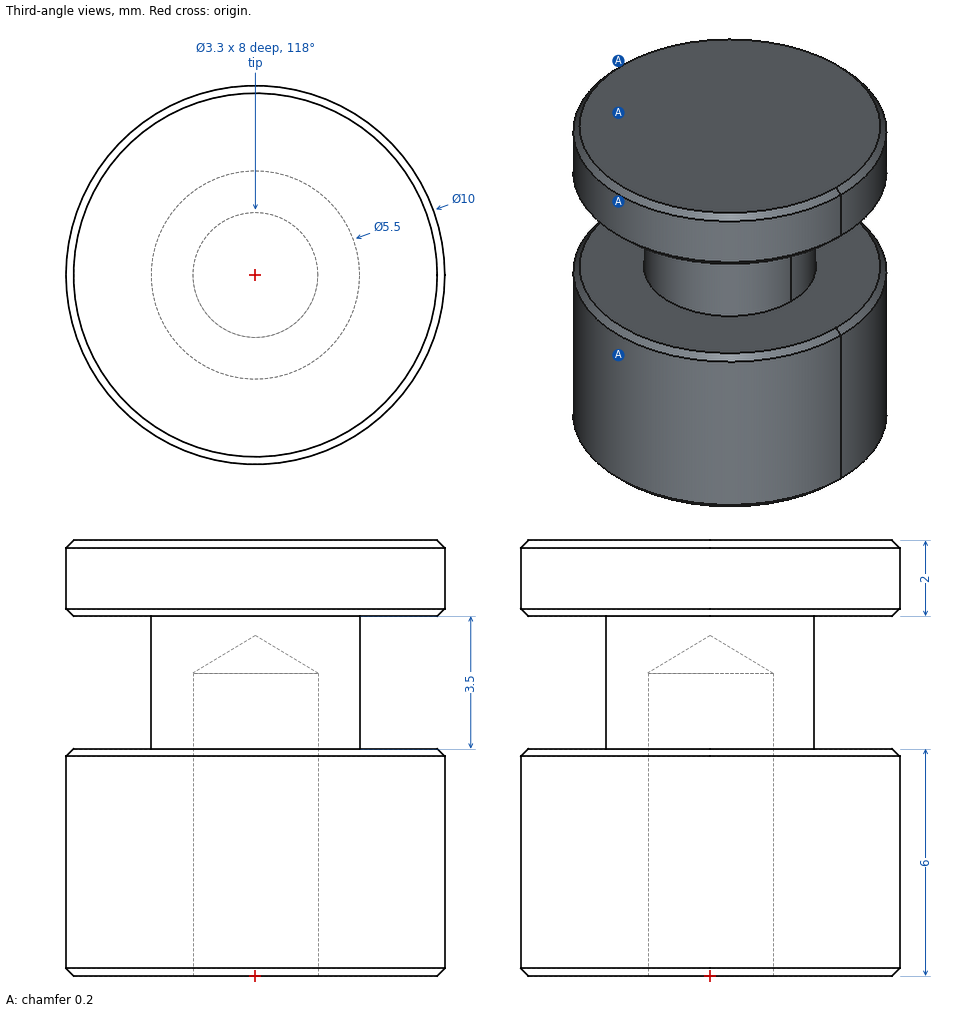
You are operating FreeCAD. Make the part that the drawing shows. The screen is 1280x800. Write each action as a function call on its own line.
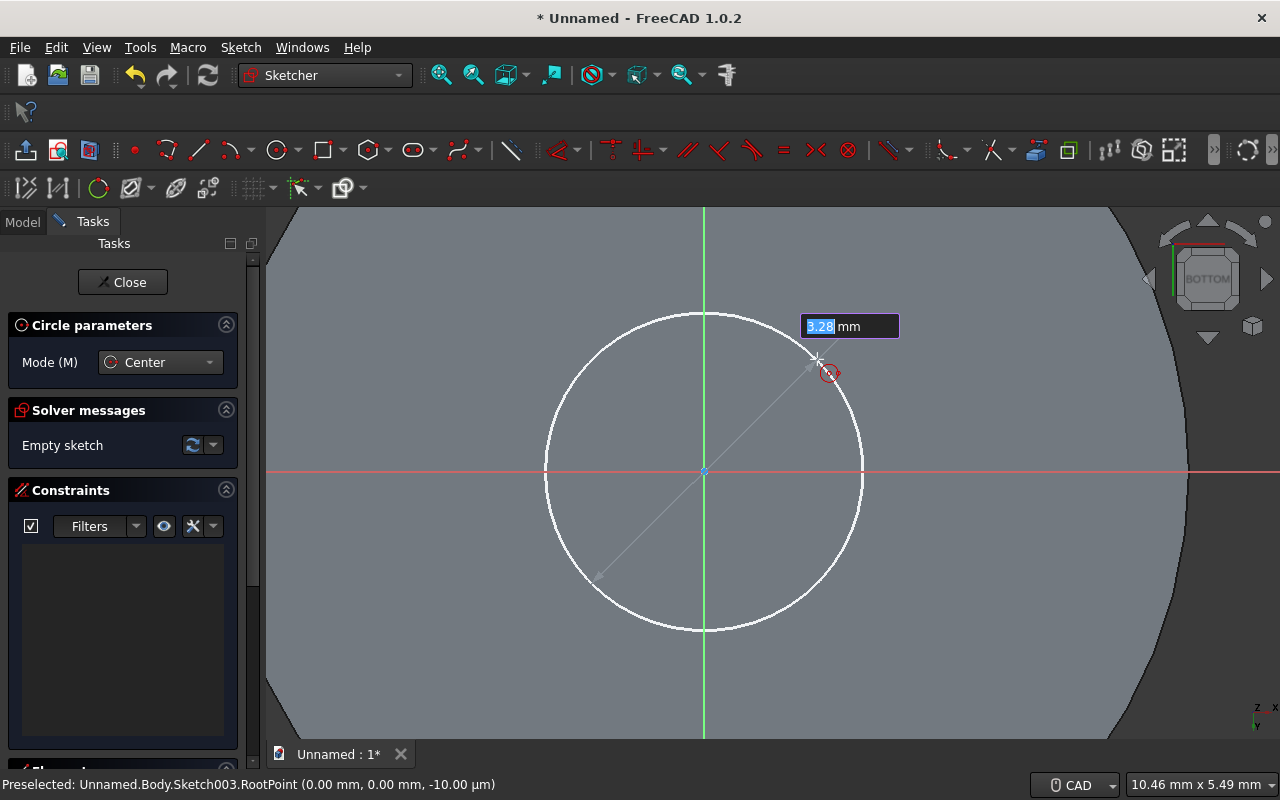
text(3.3)
key(Return)
key(Escape)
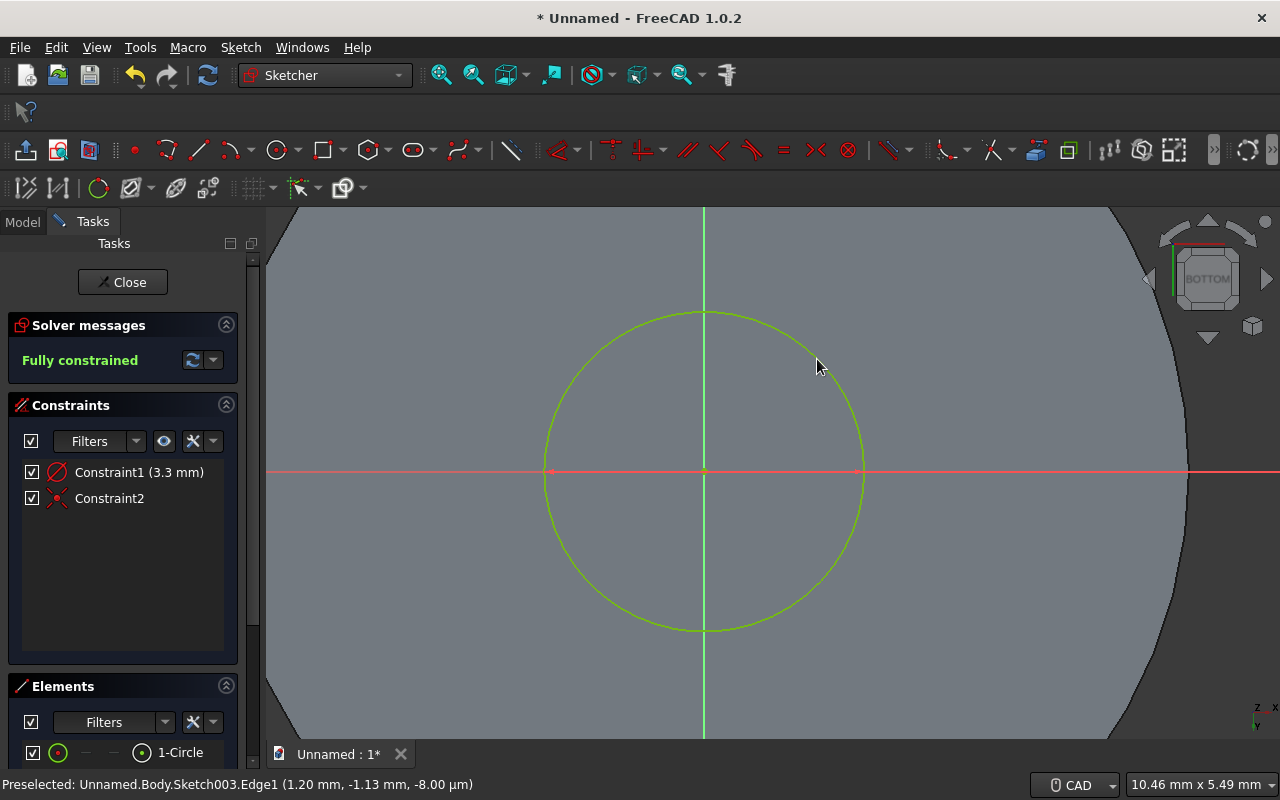
click(123, 282)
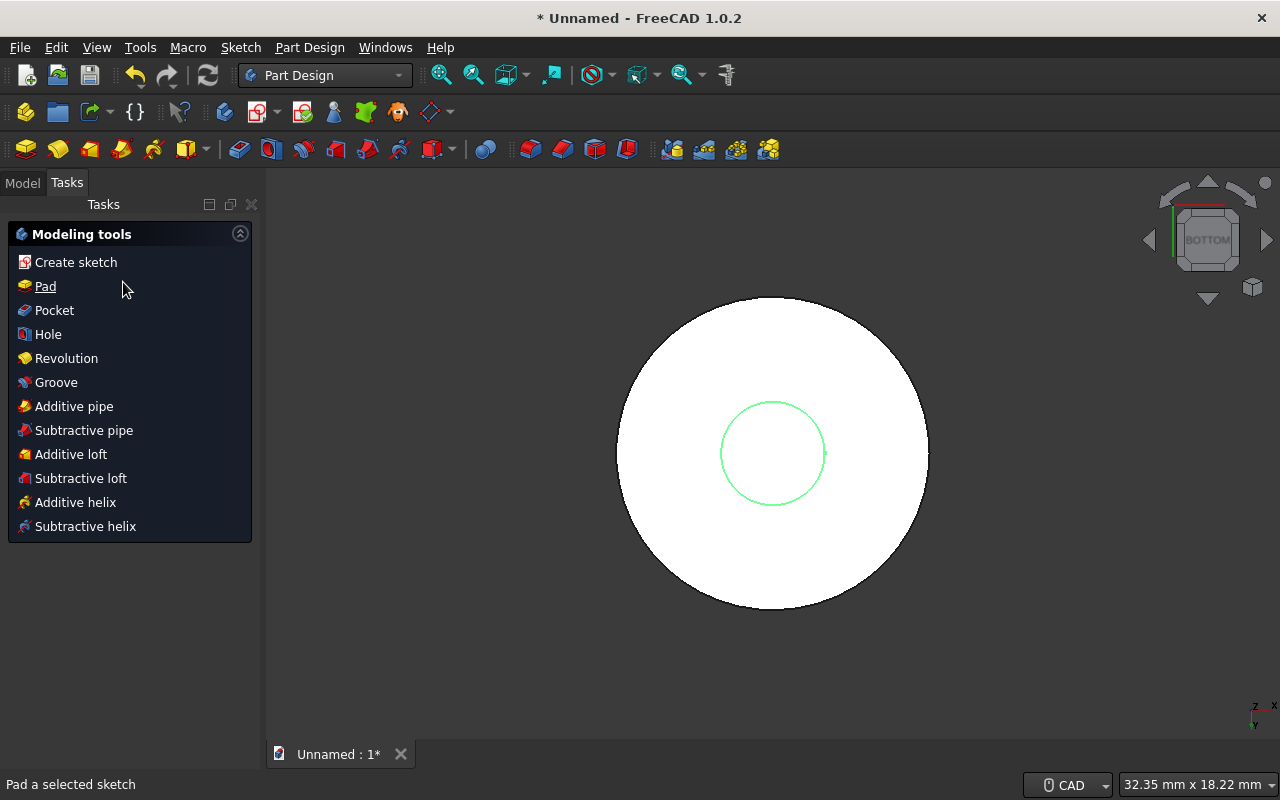
click(272, 150)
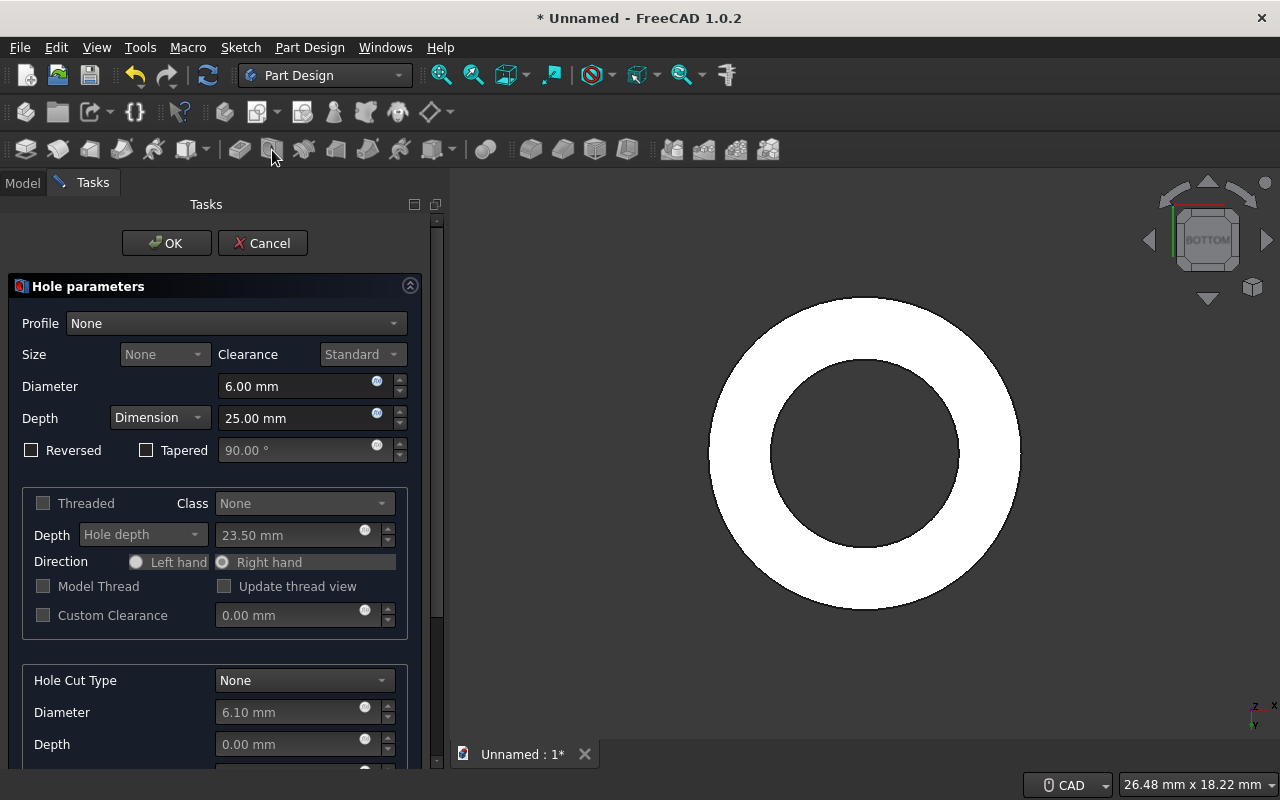
triple_click(305, 386)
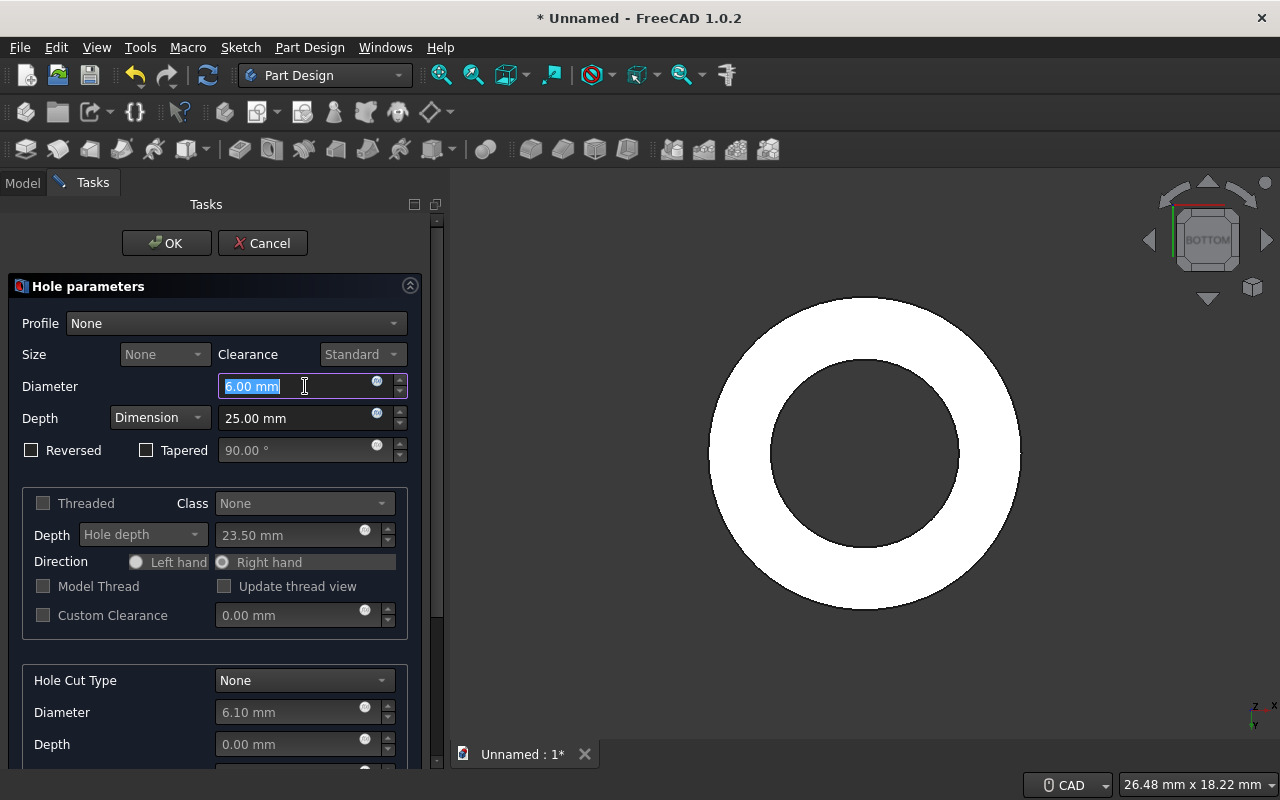
text(3.3)
key(Tab)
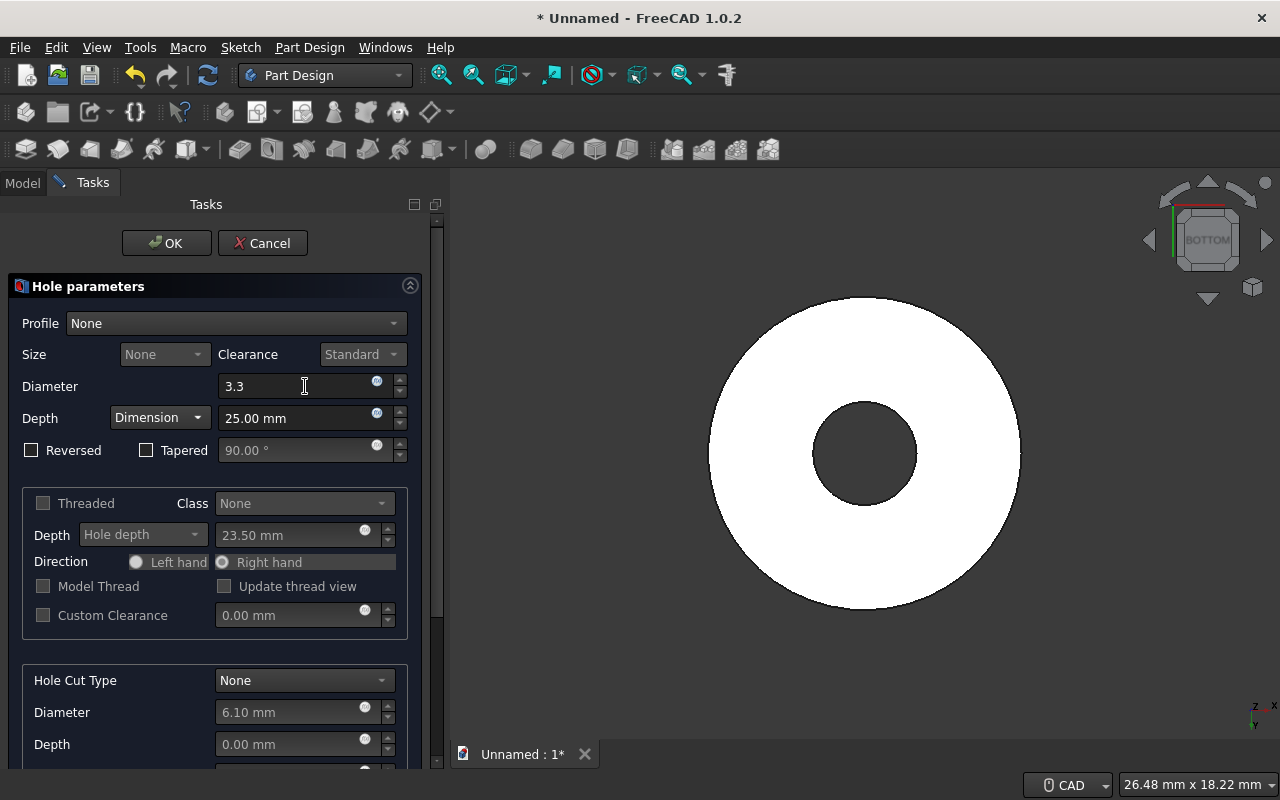
triple_click(305, 418)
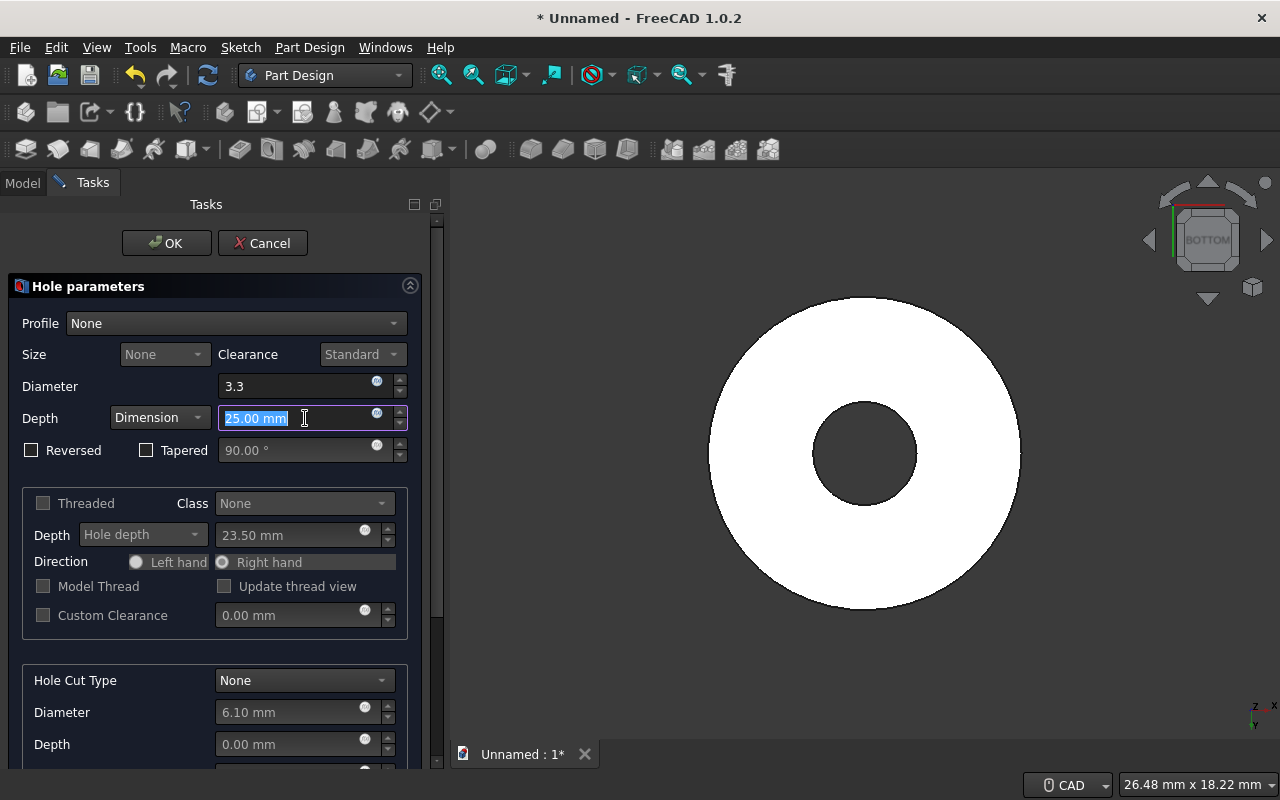
text(8)
key(Tab)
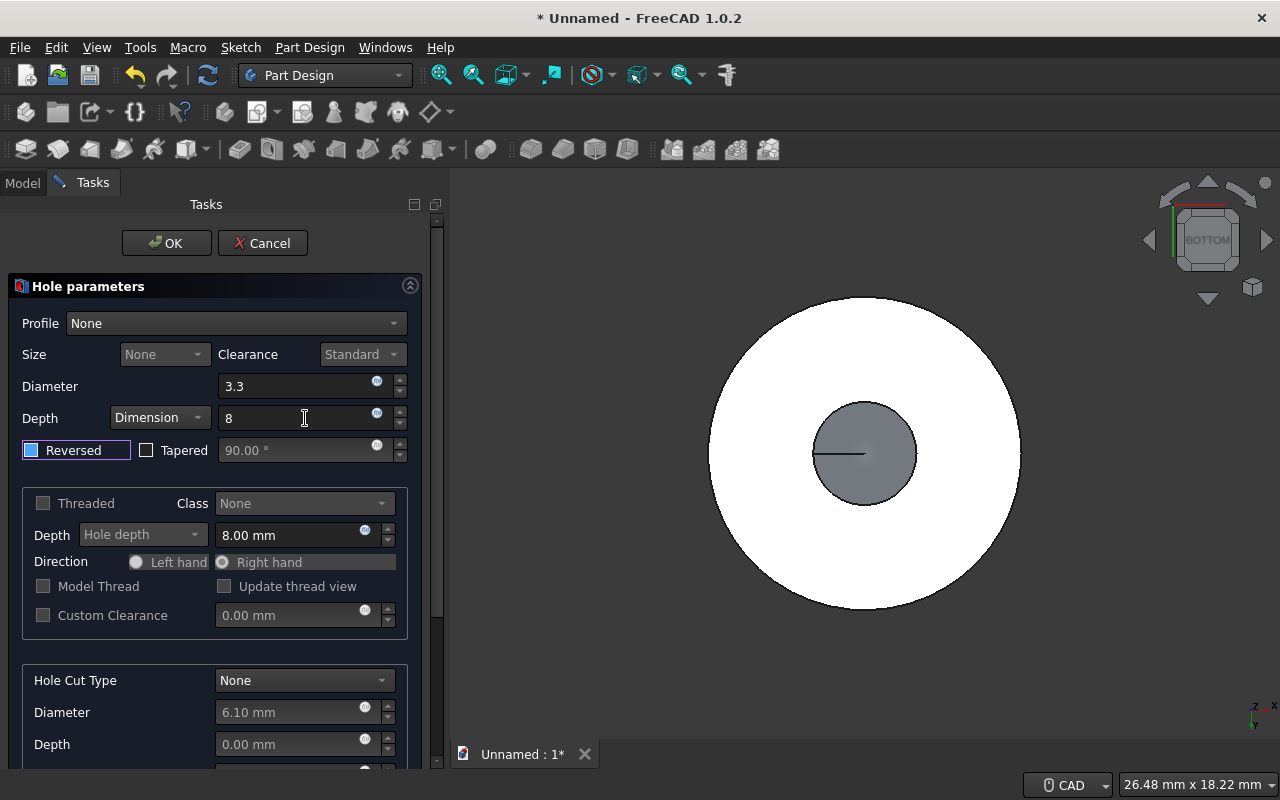
click(167, 243)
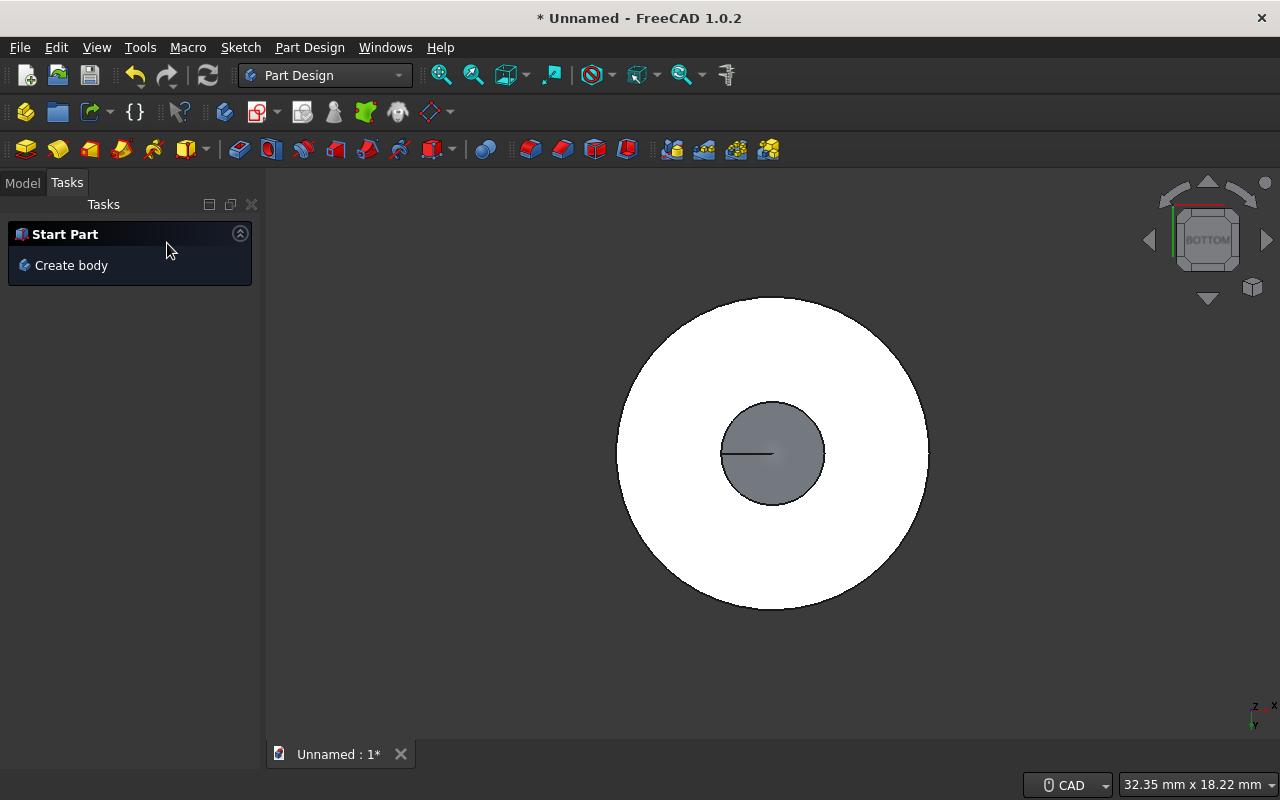
click(616, 453)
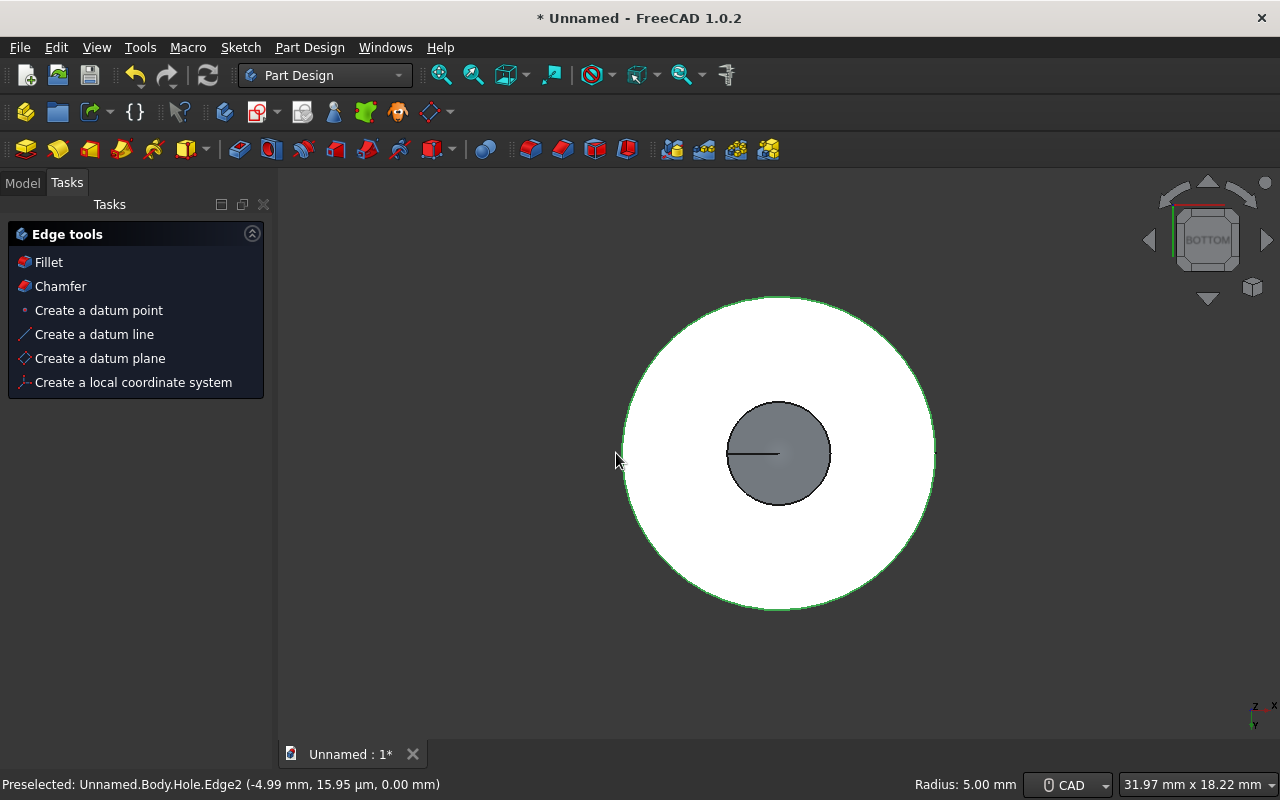
key(0)